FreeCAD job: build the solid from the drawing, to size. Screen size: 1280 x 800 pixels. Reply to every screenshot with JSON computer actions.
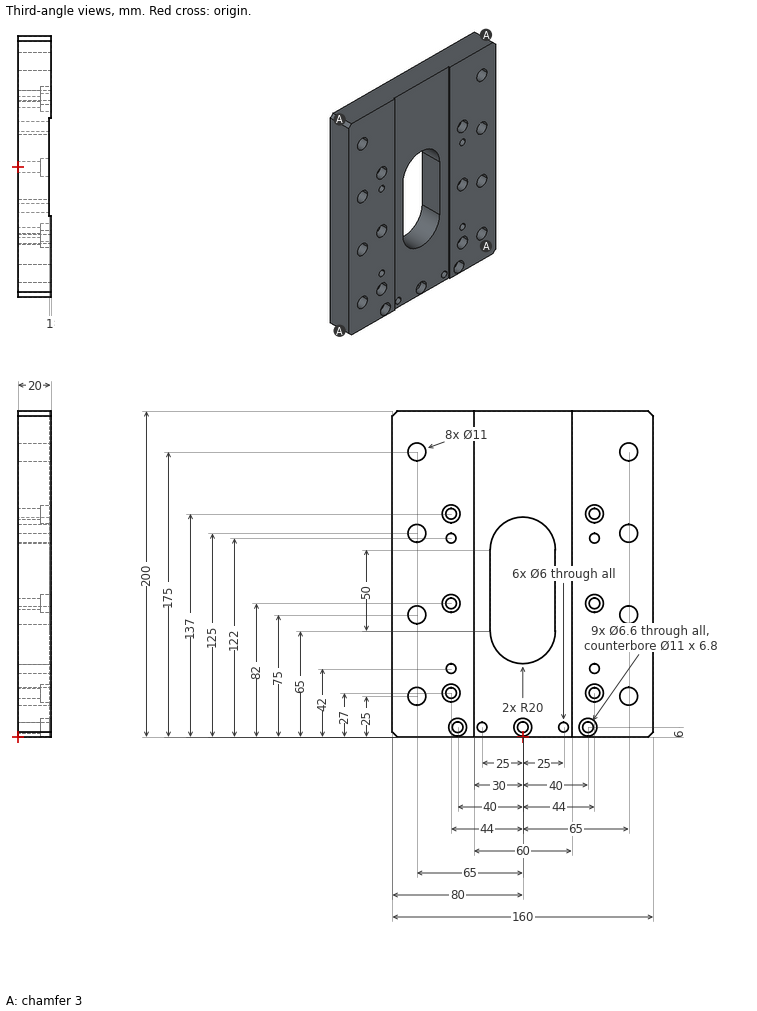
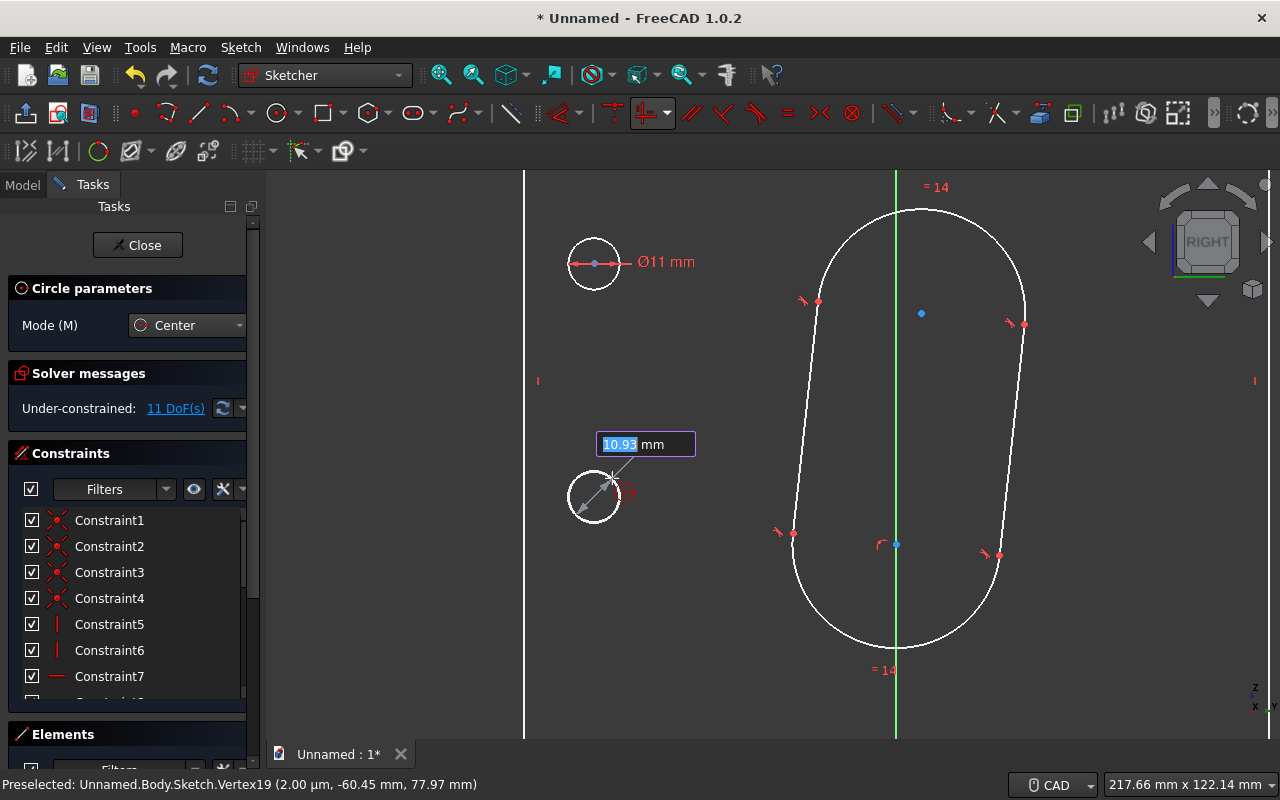
{"action": "type", "text": "11"}
{"action": "key", "text": "Return"}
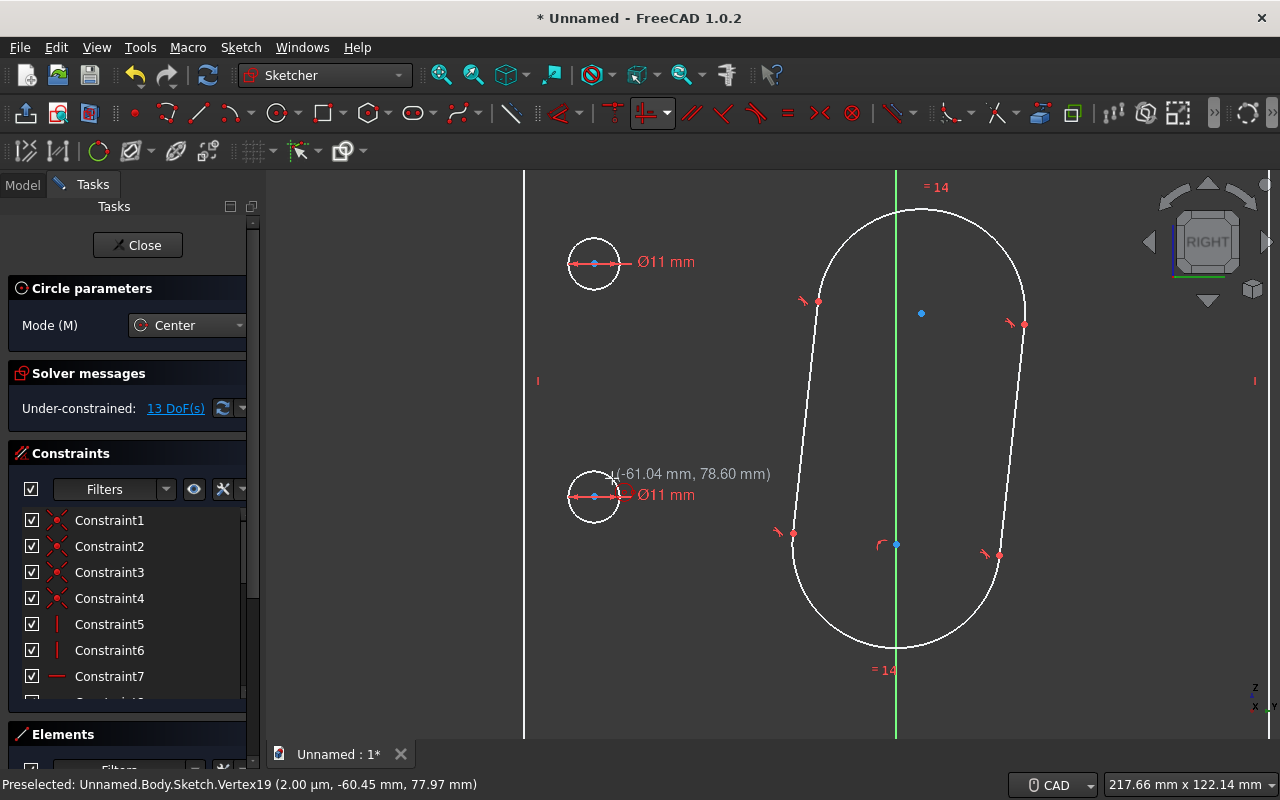
{"action": "scroll", "coordinate": [593, 498], "scroll_direction": "down", "scroll_amount": 5}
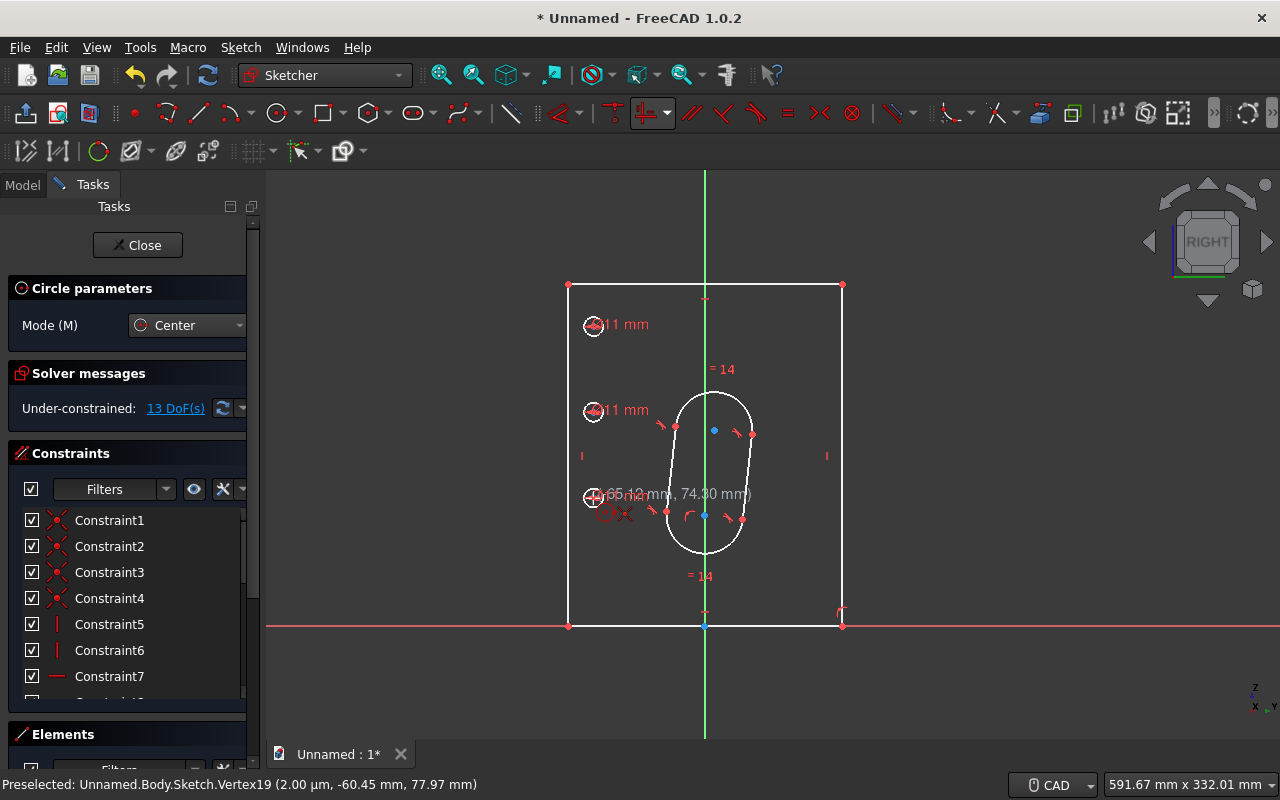
{"action": "scroll", "coordinate": [593, 583], "scroll_direction": "up", "scroll_amount": 5}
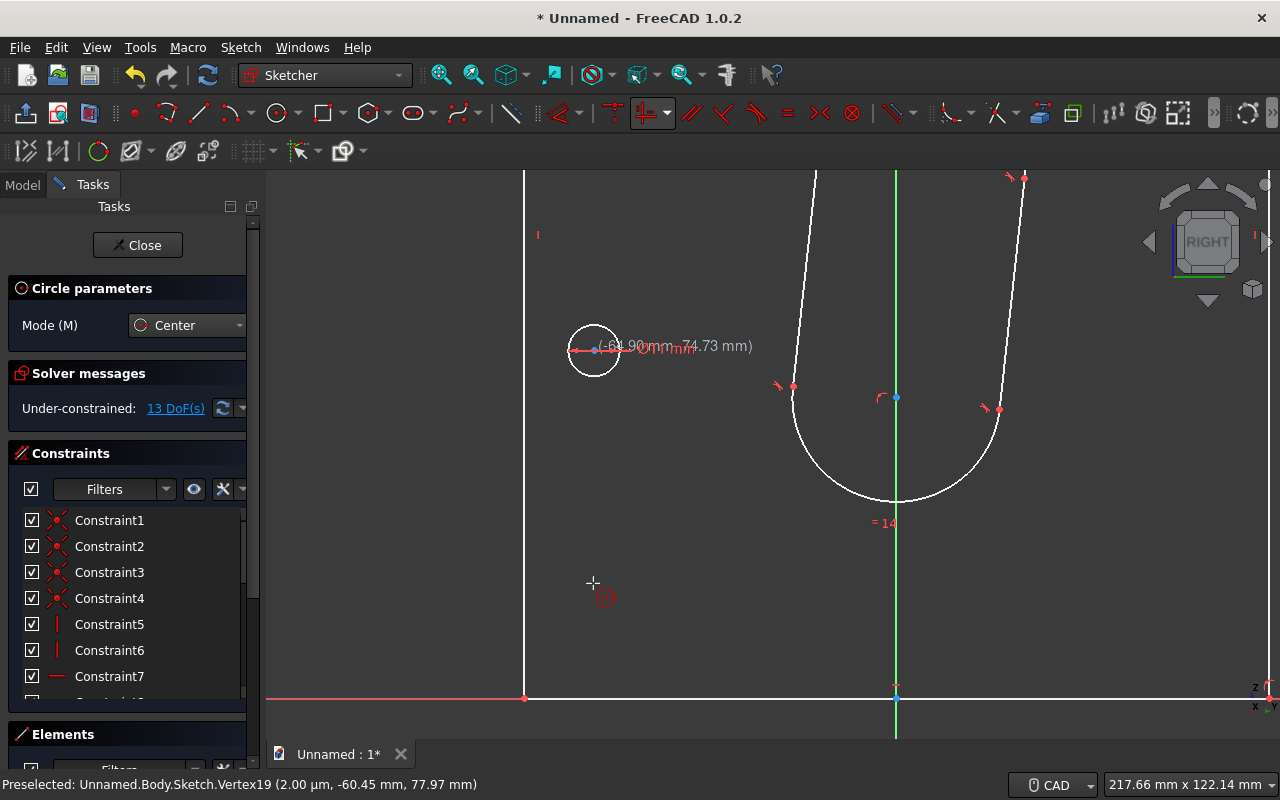
{"action": "left_click", "coordinate": [594, 582]}
{"action": "mouse_move", "coordinate": [612, 564]}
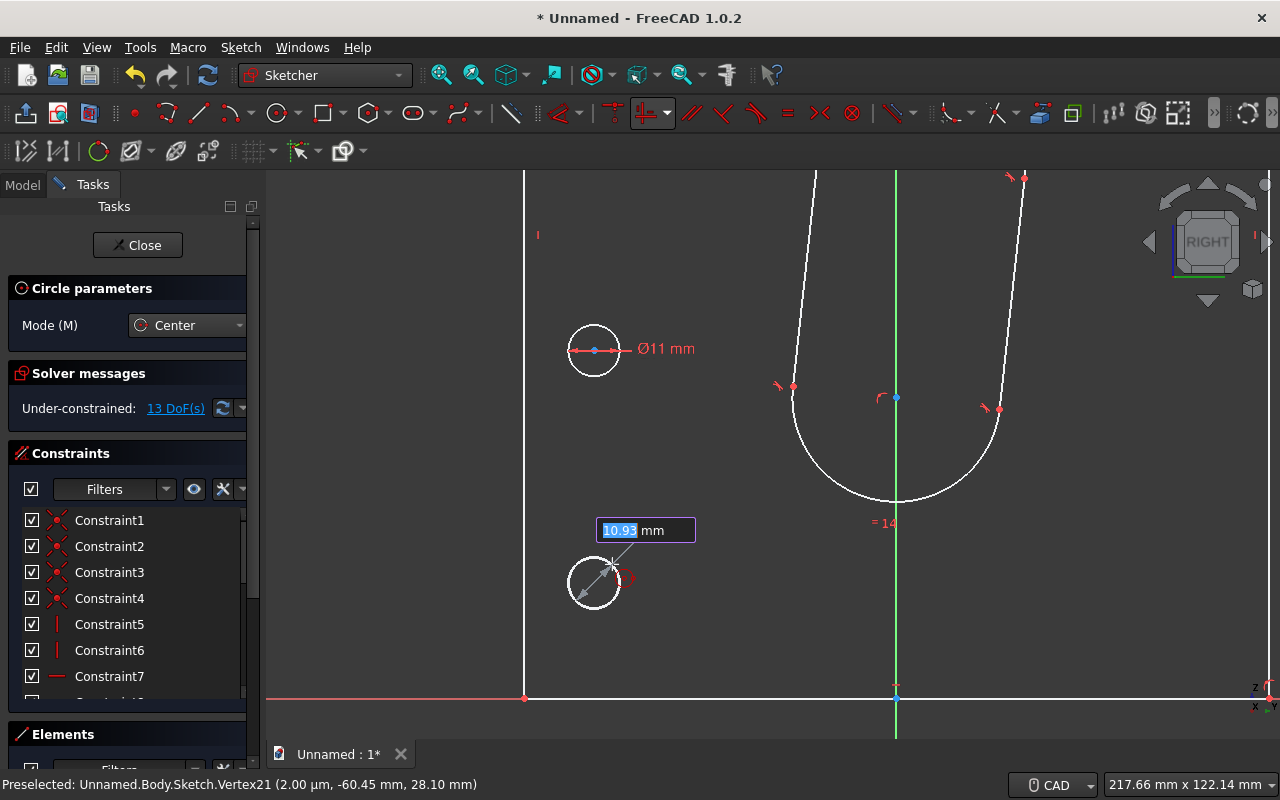
{"action": "type", "text": "11"}
{"action": "key", "text": "Return"}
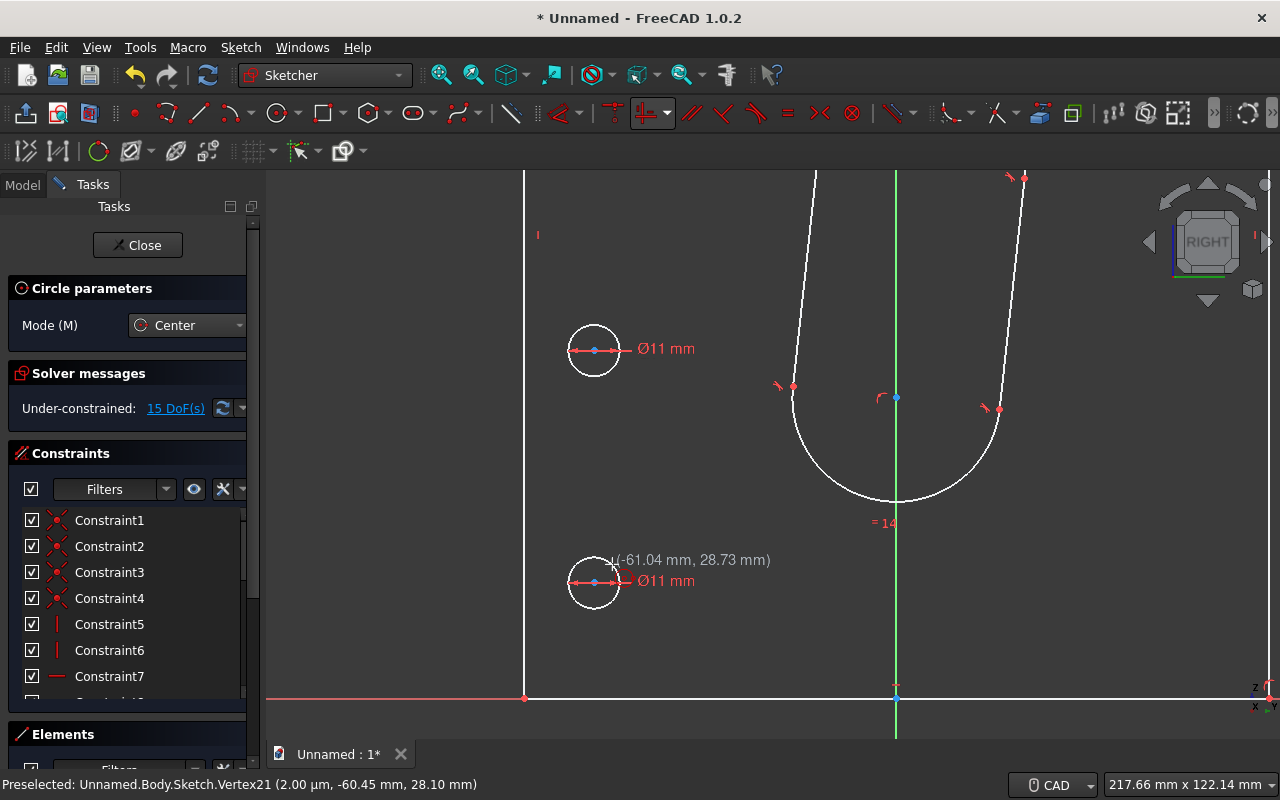
{"action": "scroll", "coordinate": [593, 583], "scroll_direction": "down", "scroll_amount": 5}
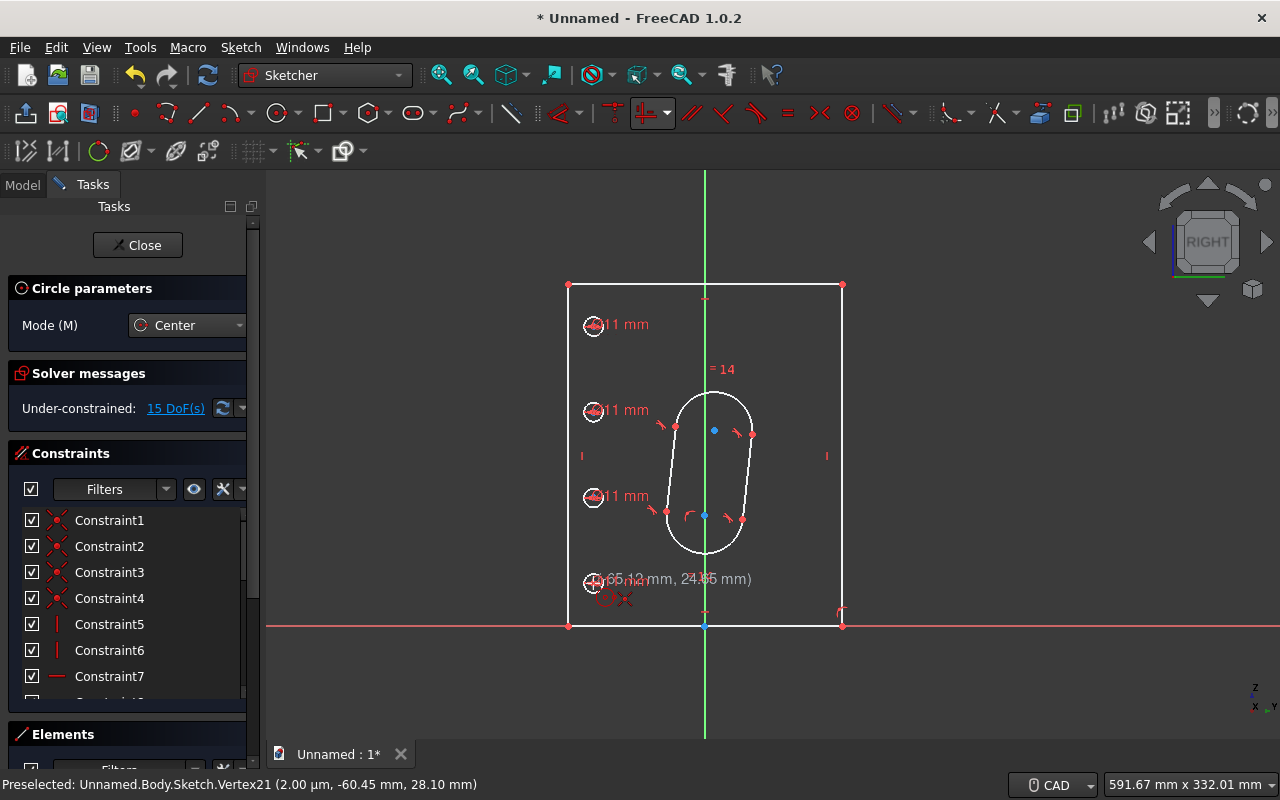
{"action": "scroll", "coordinate": [816, 326], "scroll_direction": "up", "scroll_amount": 5}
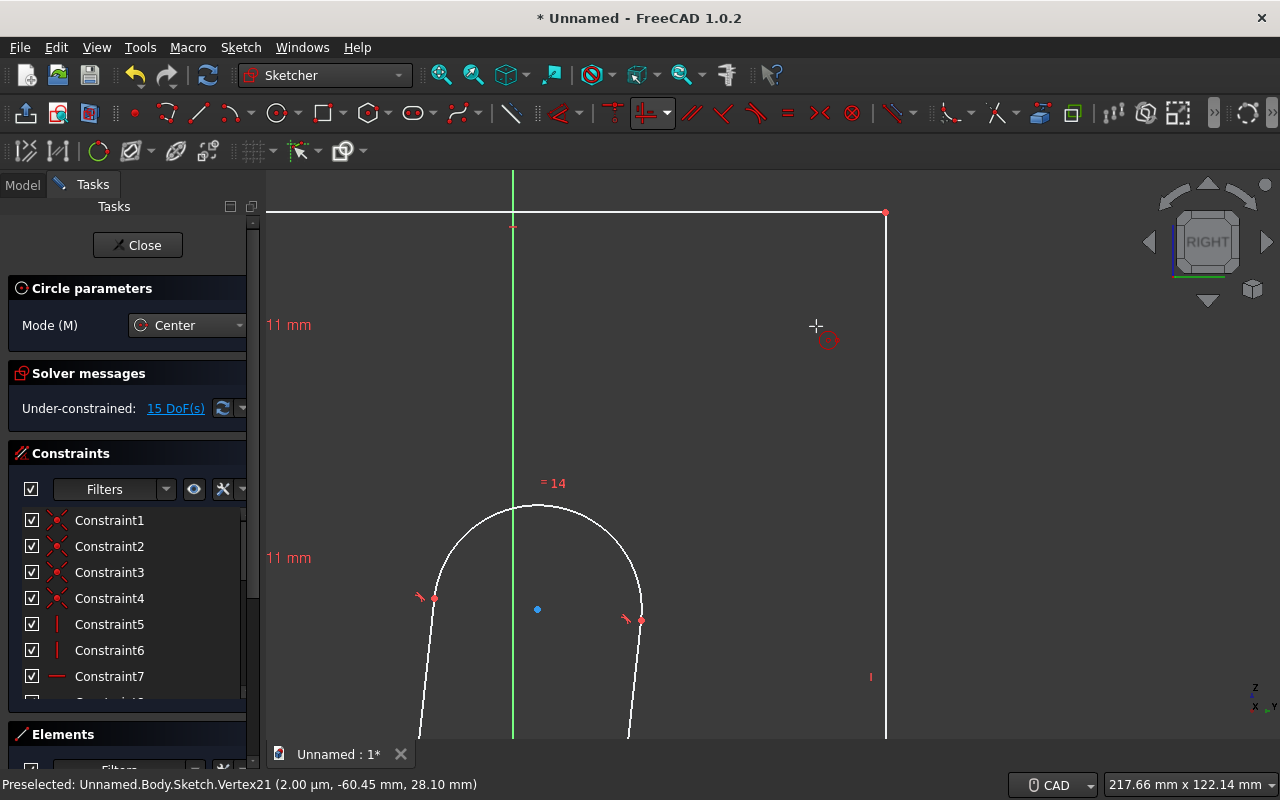
{"action": "left_click", "coordinate": [816, 326]}
{"action": "mouse_move", "coordinate": [834, 308]}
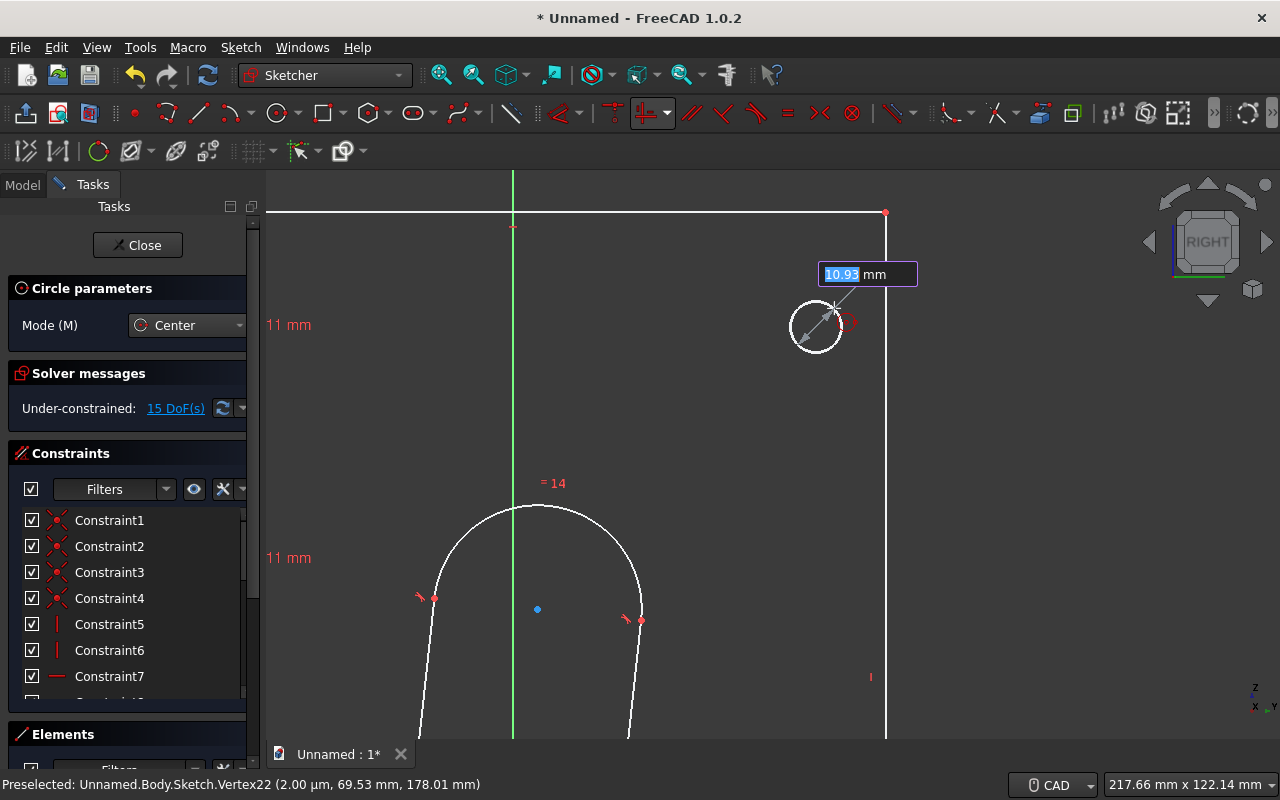
{"action": "type", "text": "11"}
{"action": "key", "text": "Return"}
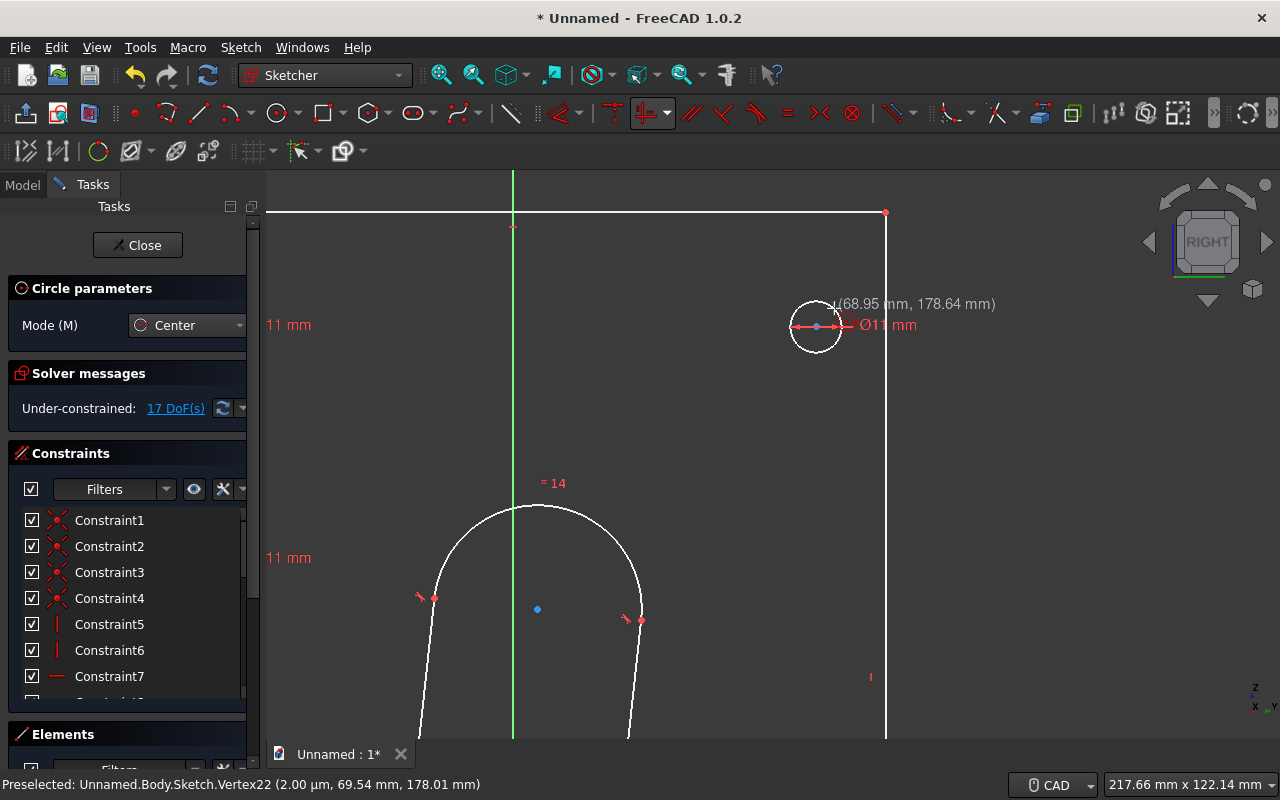
{"action": "left_click", "coordinate": [816, 559]}
{"action": "mouse_move", "coordinate": [834, 541]}